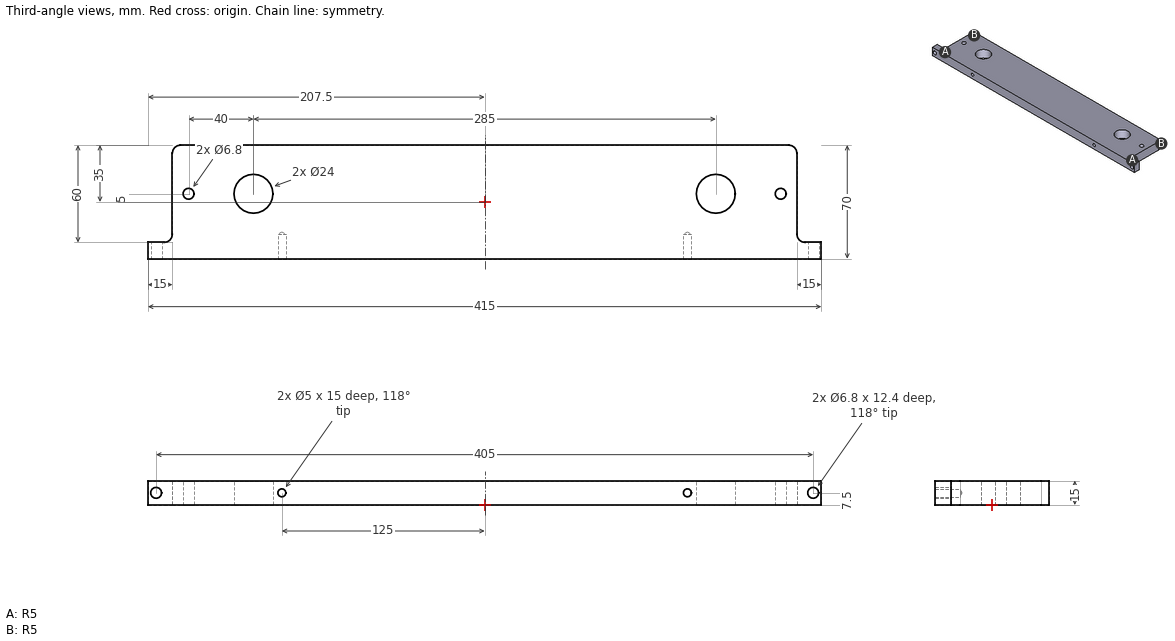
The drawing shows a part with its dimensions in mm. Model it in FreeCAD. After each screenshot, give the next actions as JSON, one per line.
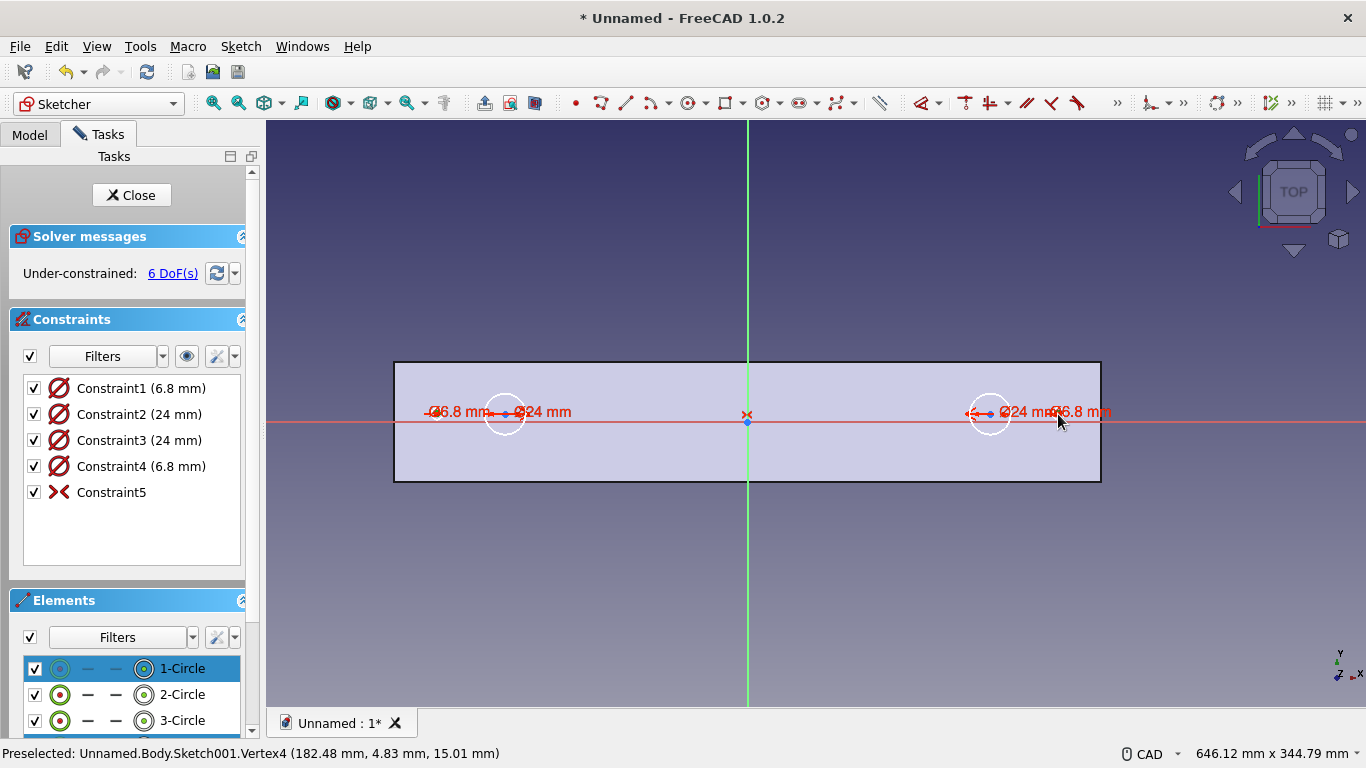
{"action": "left_click", "coordinate": [748, 641]}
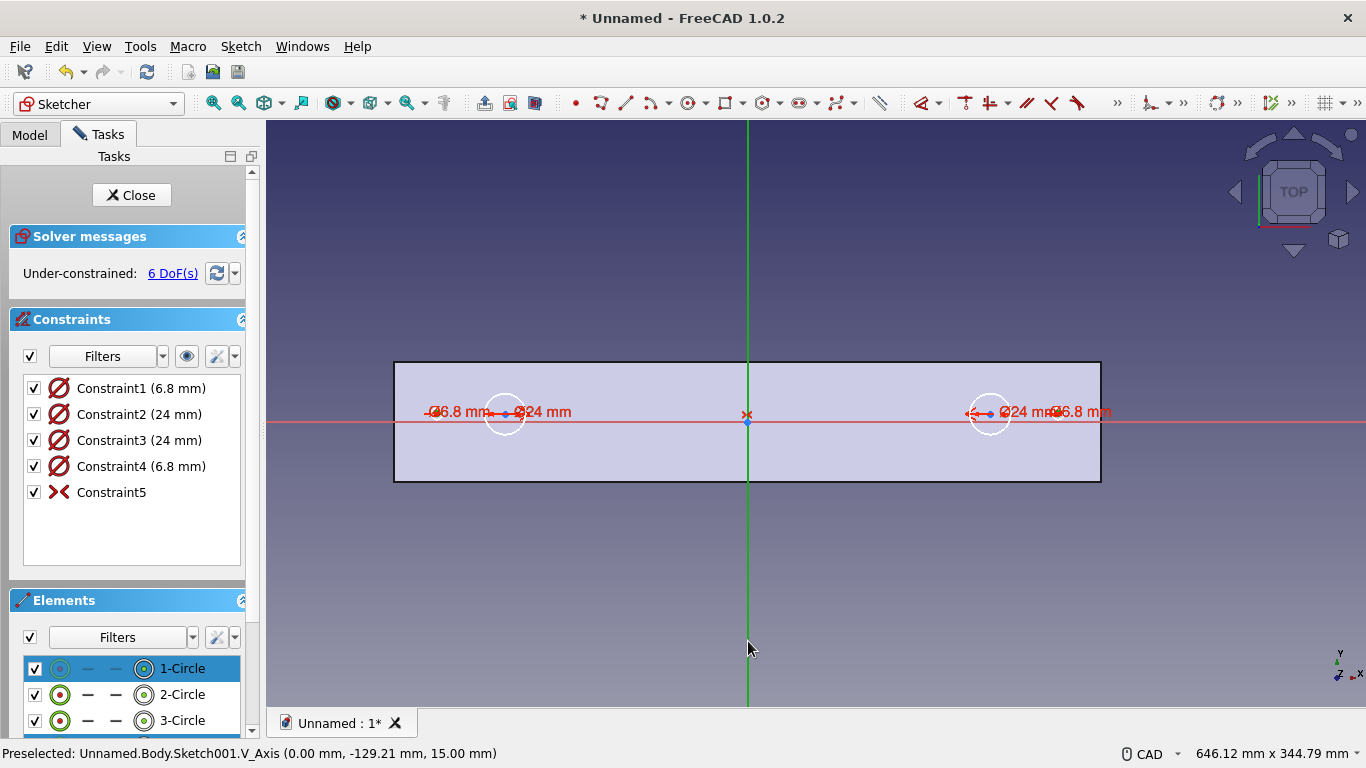
{"action": "key", "text": "s"}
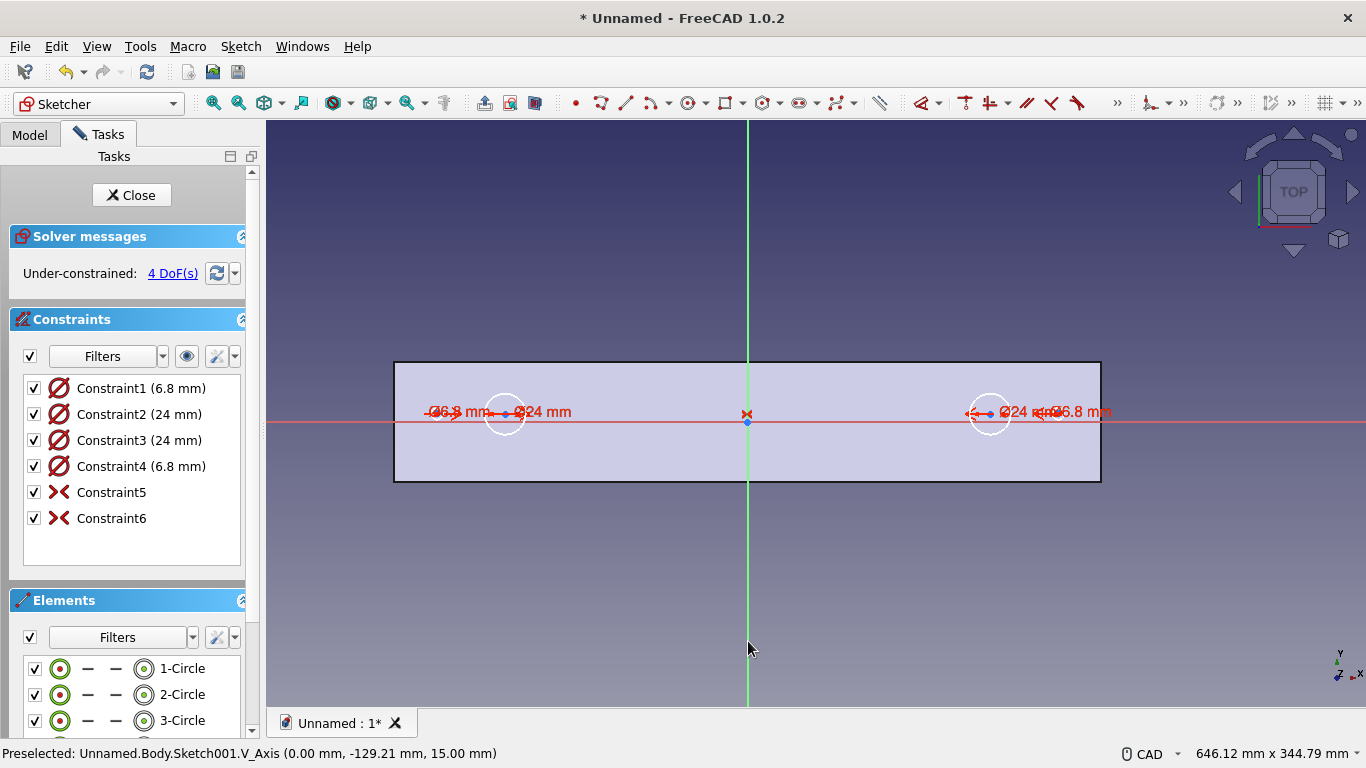
{"action": "left_click", "coordinate": [920, 104]}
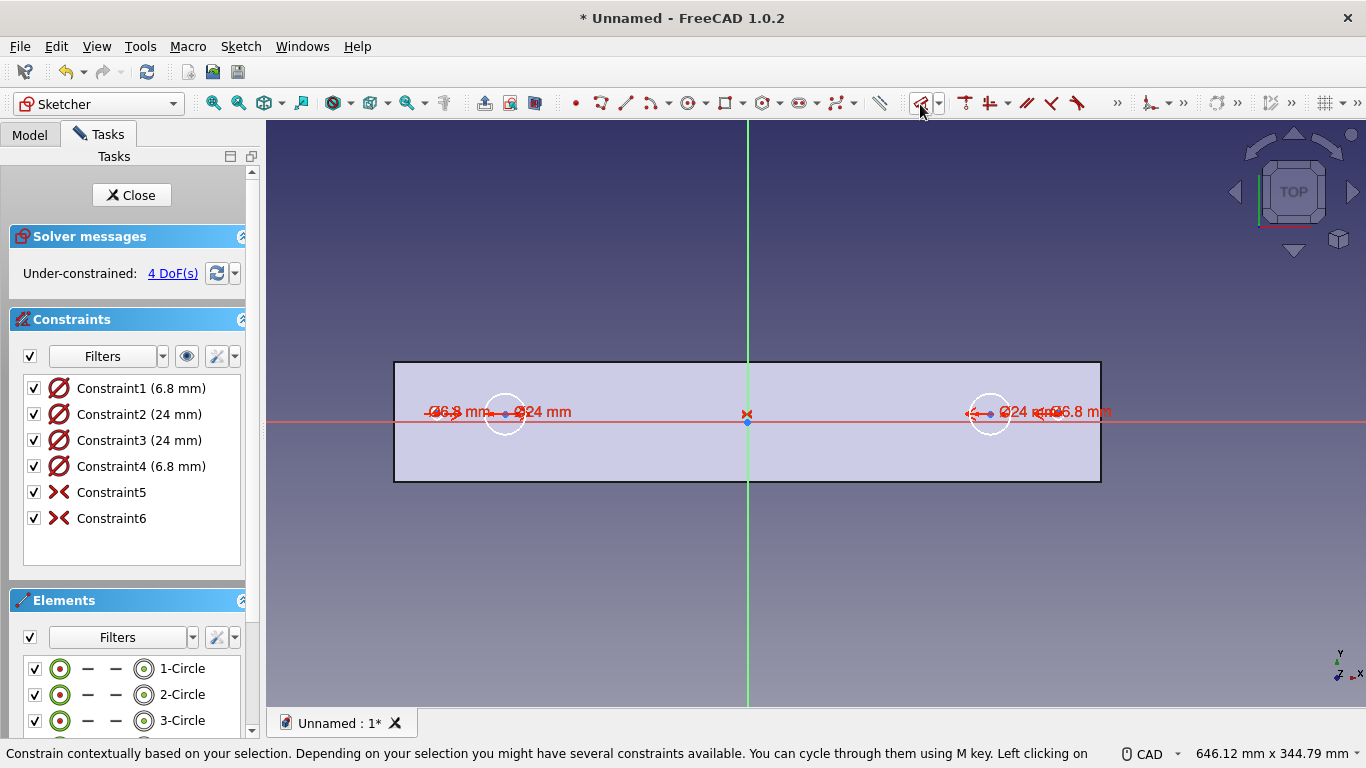
{"action": "scroll", "coordinate": [437, 414], "scroll_direction": "up", "scroll_amount": 8}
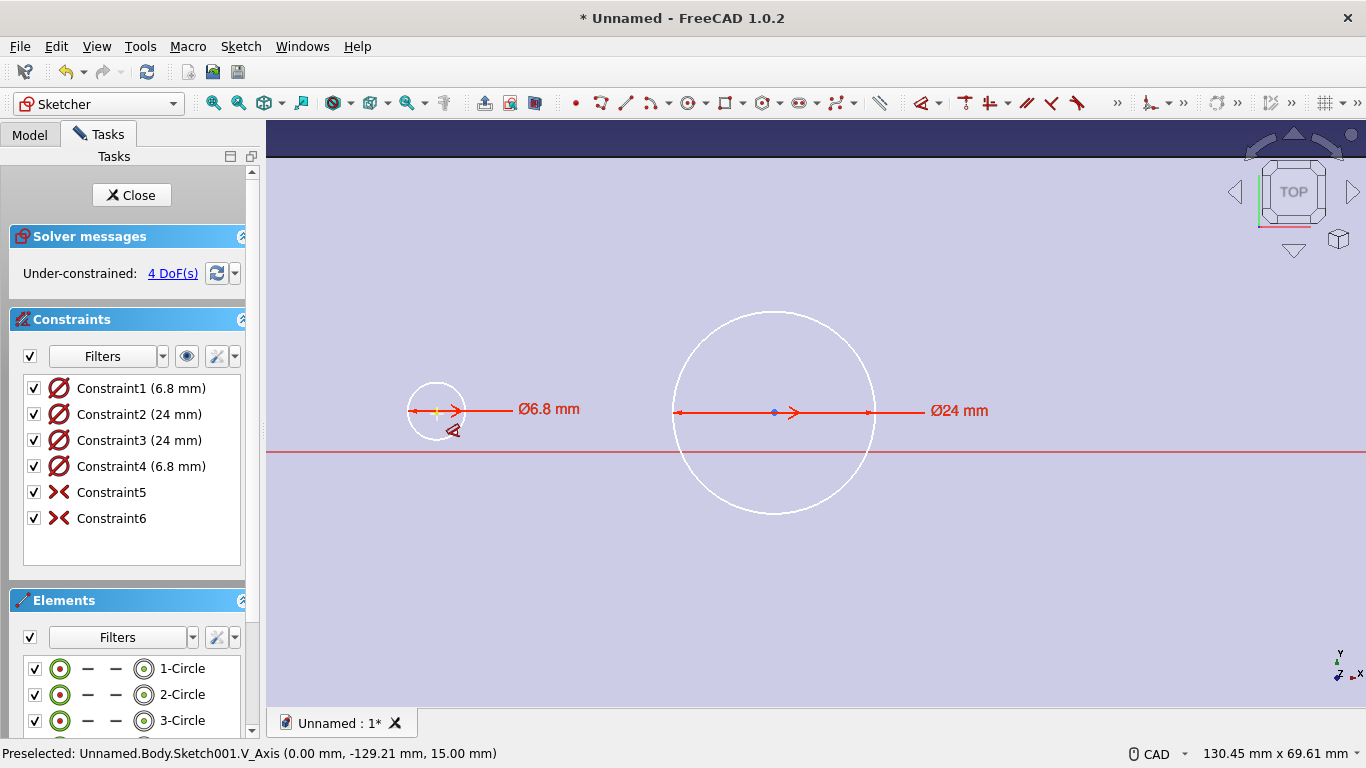
{"action": "left_click", "coordinate": [437, 411]}
{"action": "left_click", "coordinate": [379, 431]}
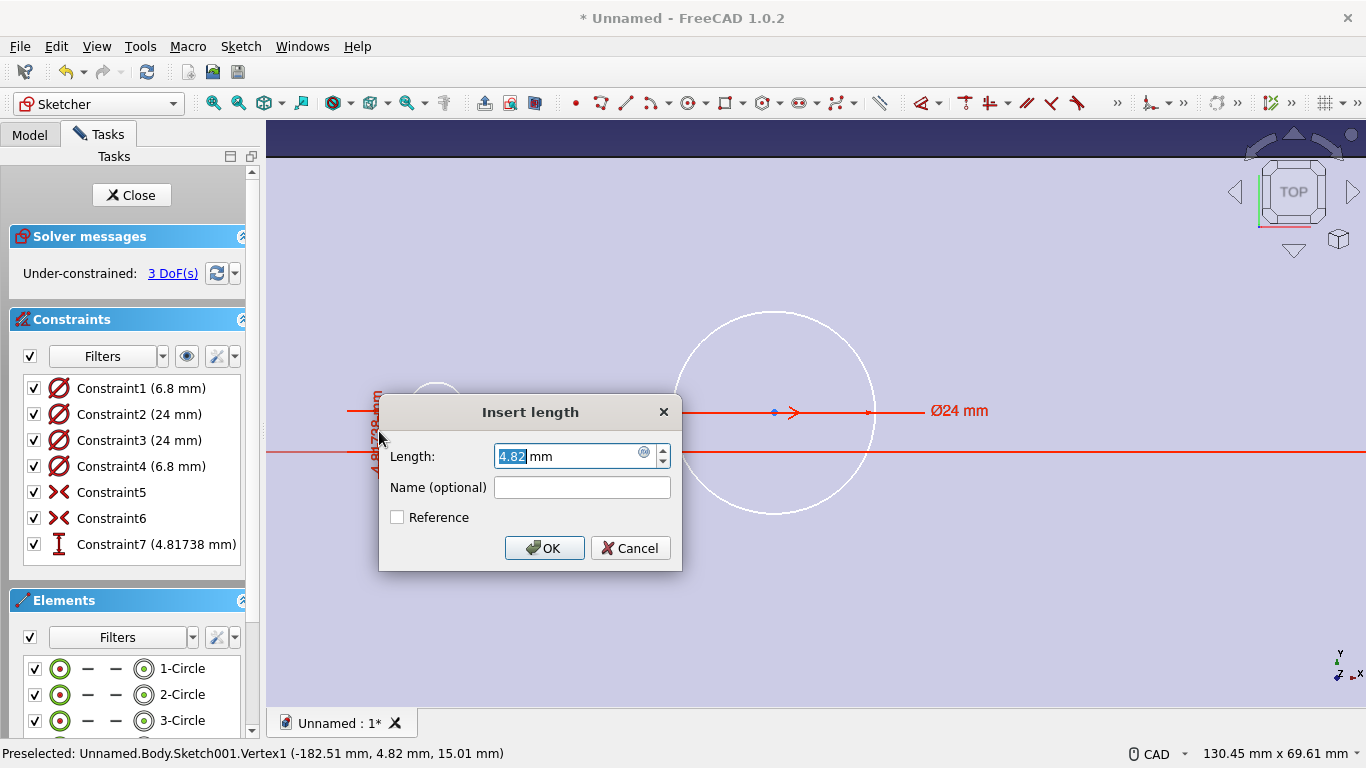
{"action": "type", "text": "5"}
{"action": "key", "text": "Return"}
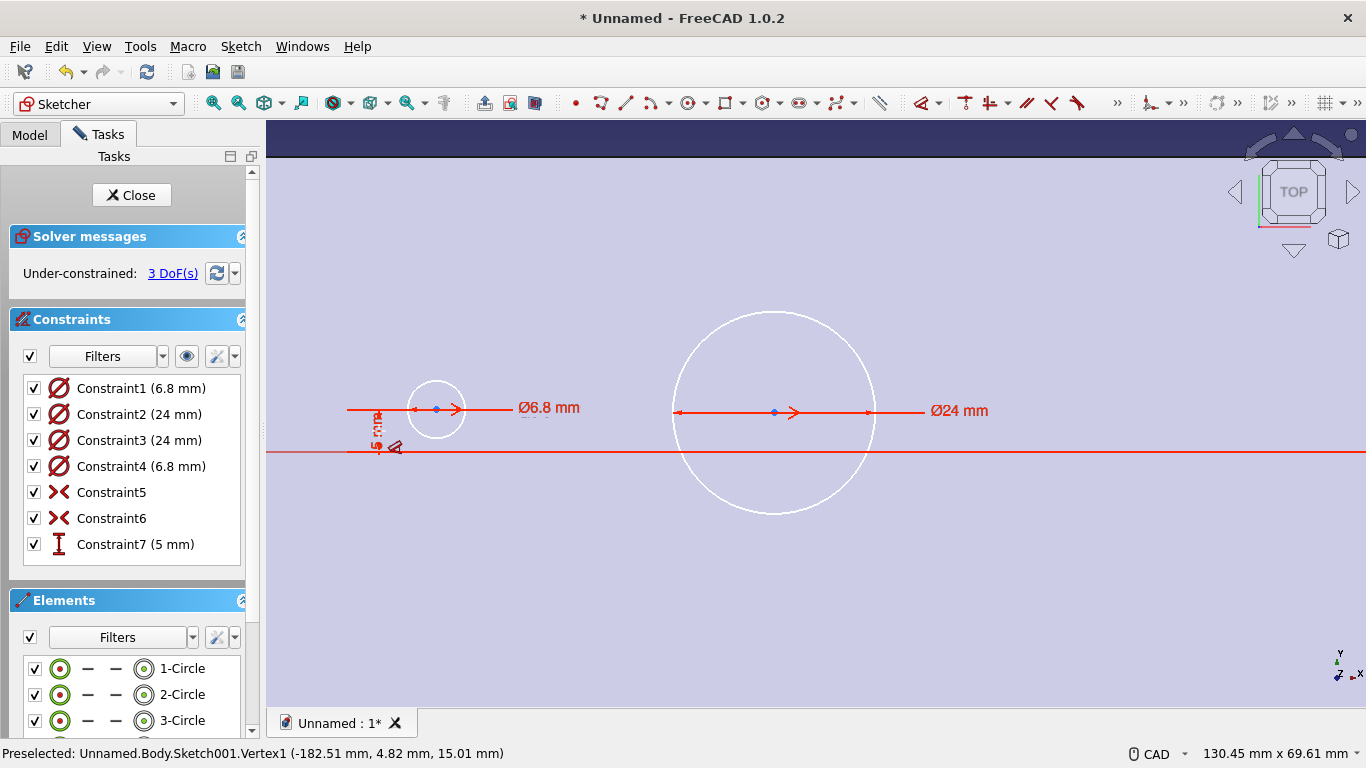
{"action": "left_click", "coordinate": [774, 413]}
{"action": "left_click", "coordinate": [740, 432]}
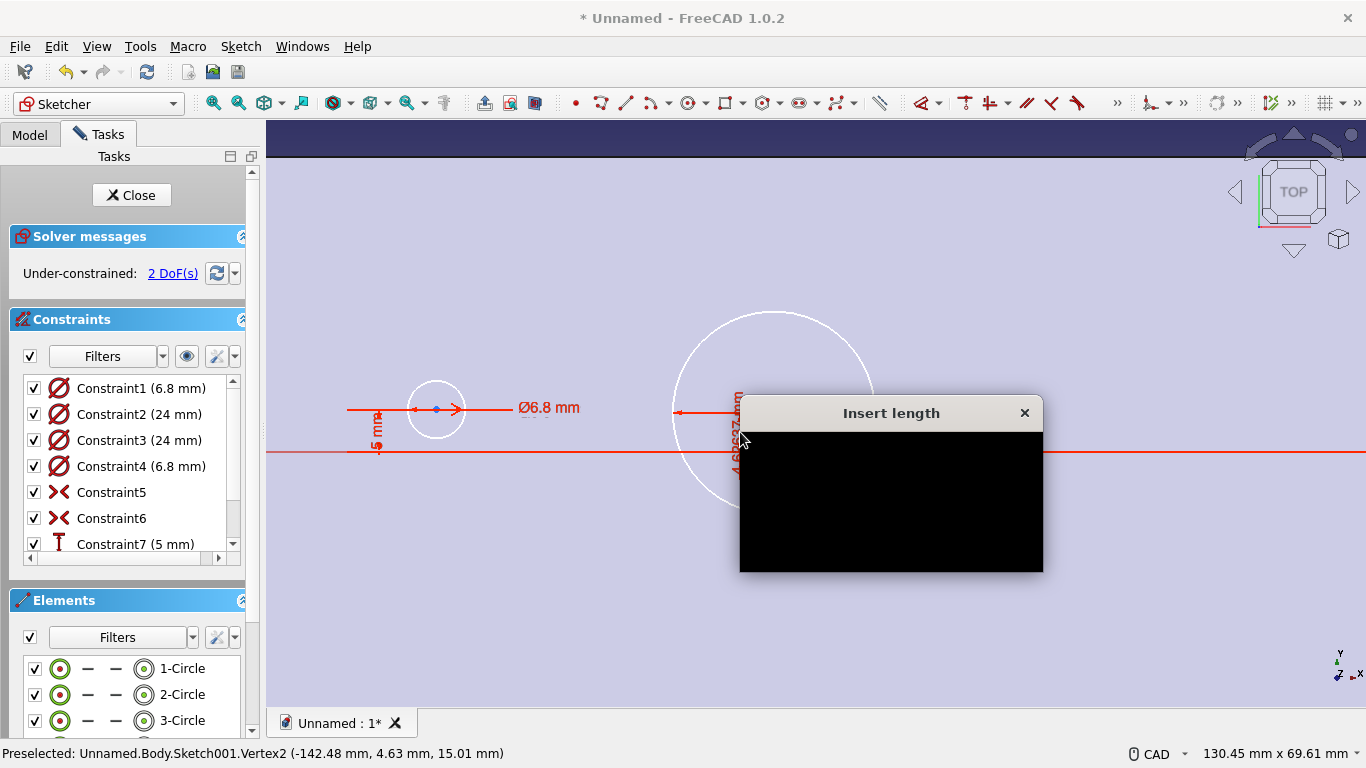
{"action": "type", "text": "5"}
{"action": "key", "text": "Return"}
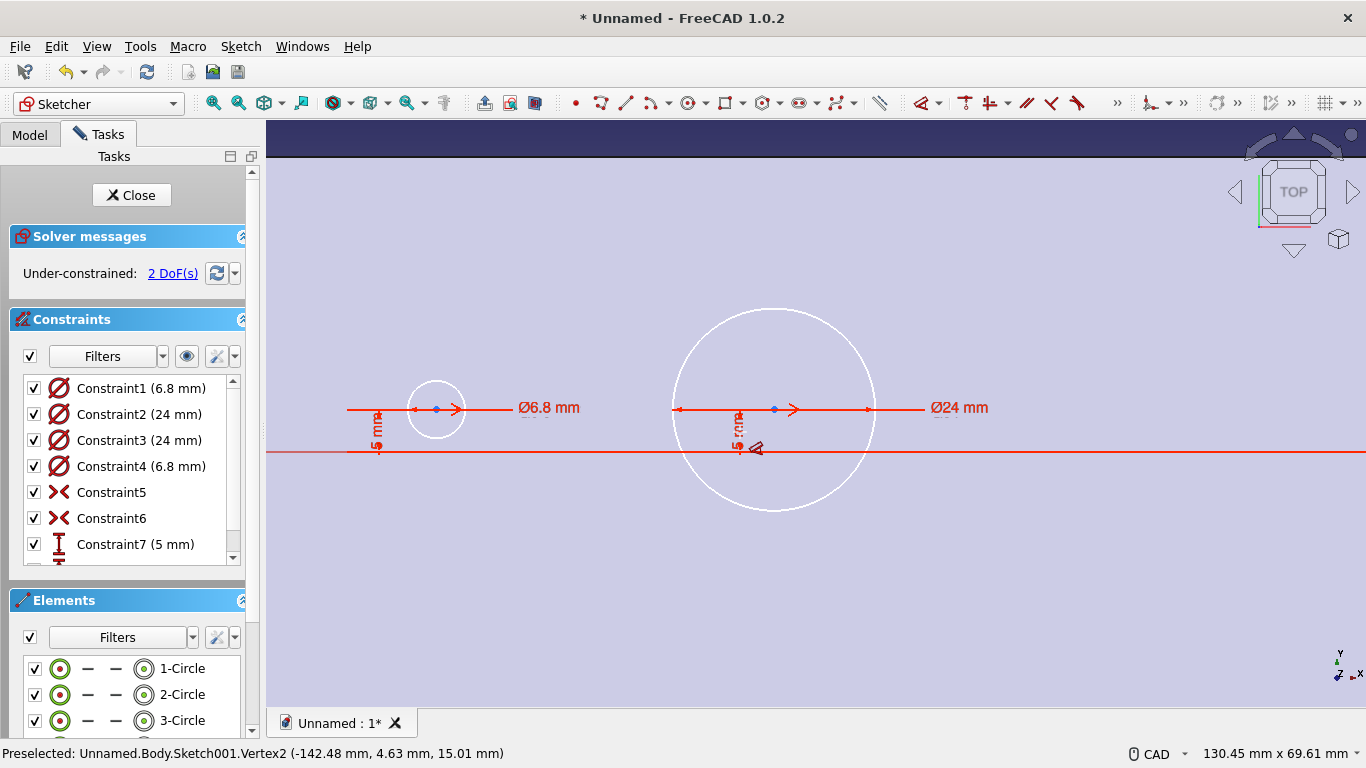
{"action": "scroll", "coordinate": [437, 414], "scroll_direction": "down", "scroll_amount": 8}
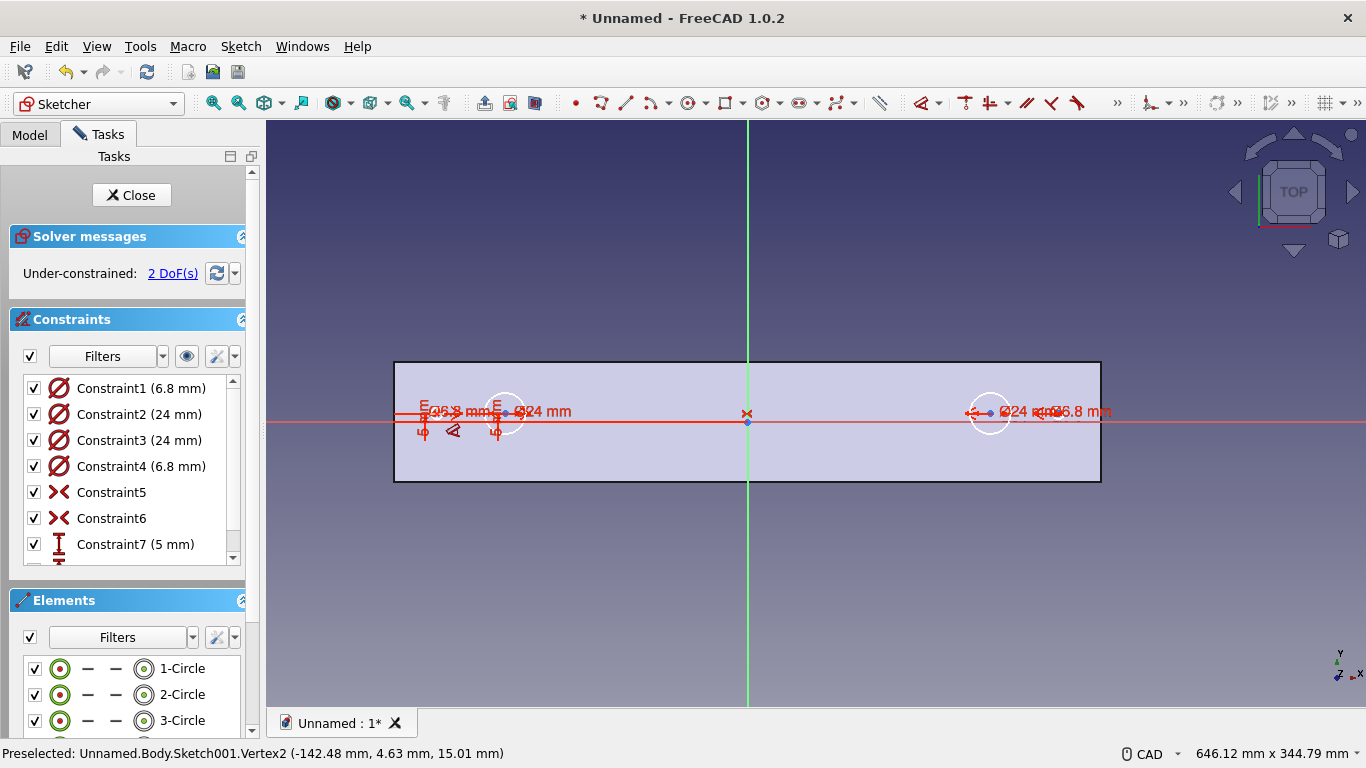
{"action": "left_click", "coordinate": [437, 414]}